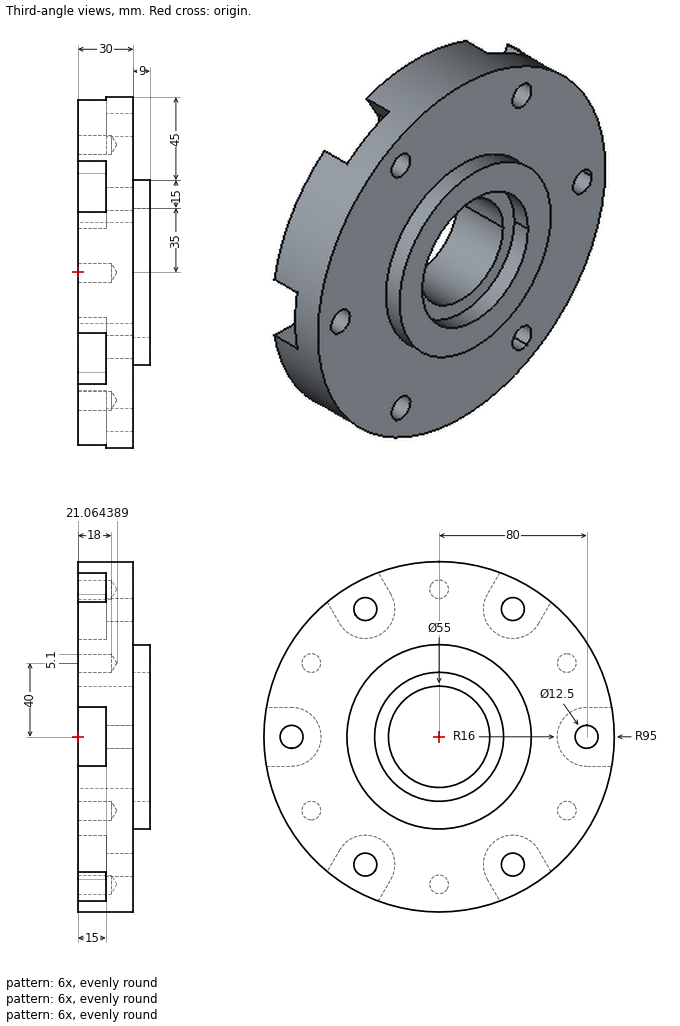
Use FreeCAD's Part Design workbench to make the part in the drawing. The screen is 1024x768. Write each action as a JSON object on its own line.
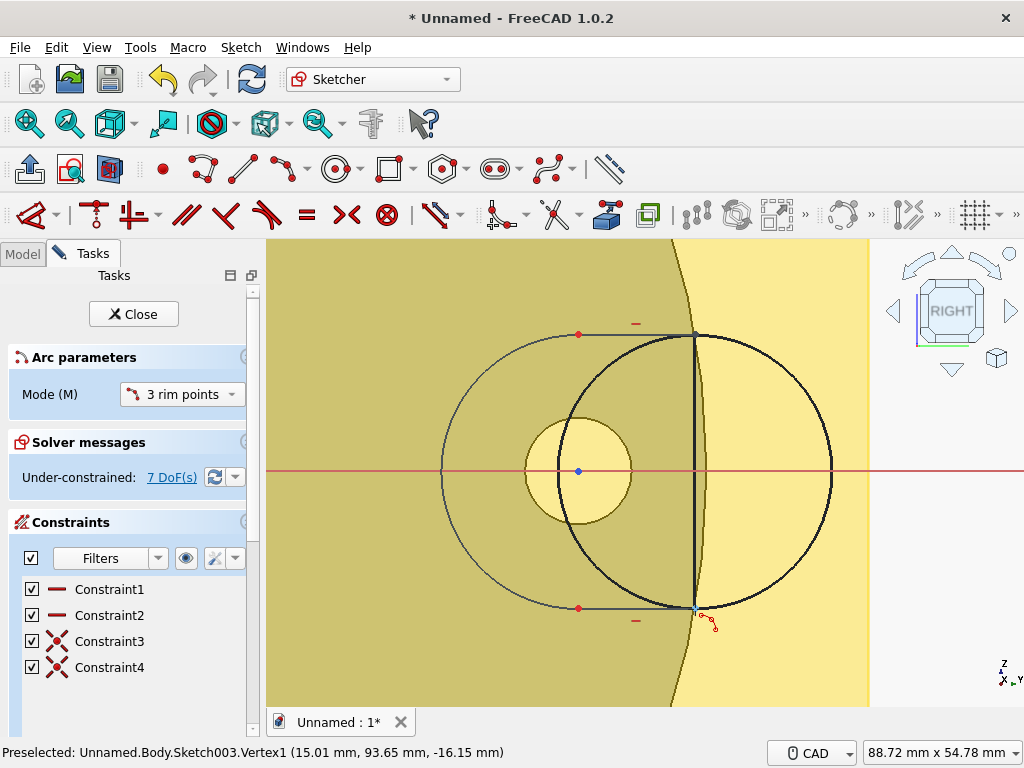
{"action": "scroll", "coordinate": [706, 498], "scroll_direction": "up", "scroll_amount": 2}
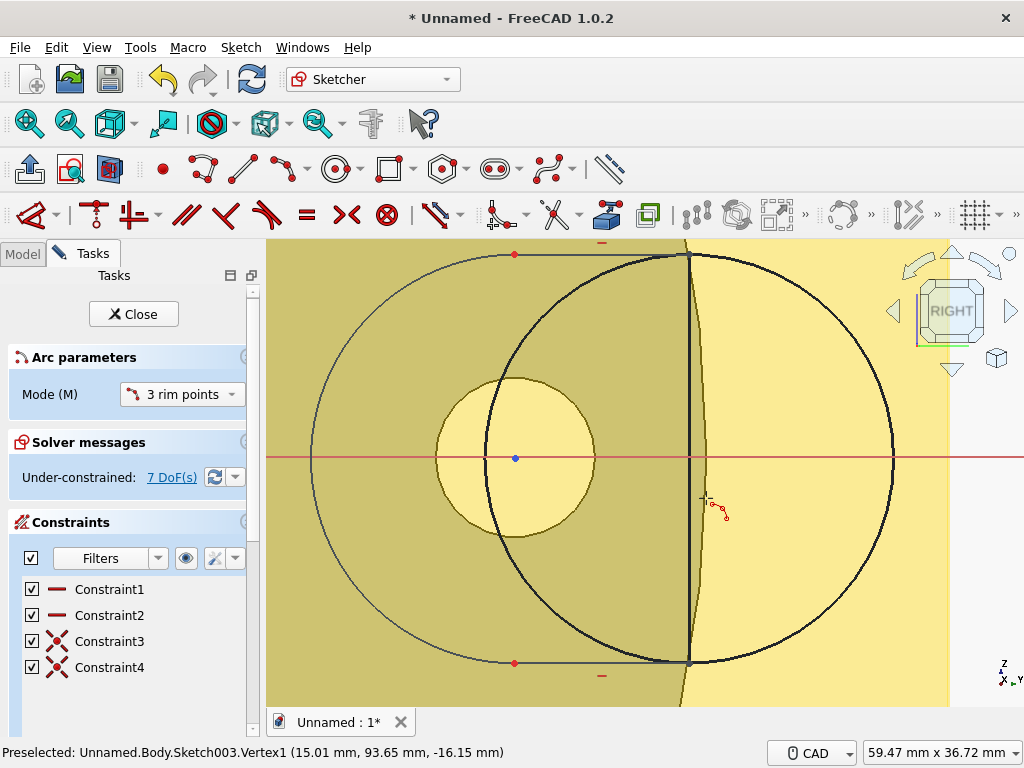
{"action": "left_click", "coordinate": [706, 498]}
{"action": "key", "text": "Escape"}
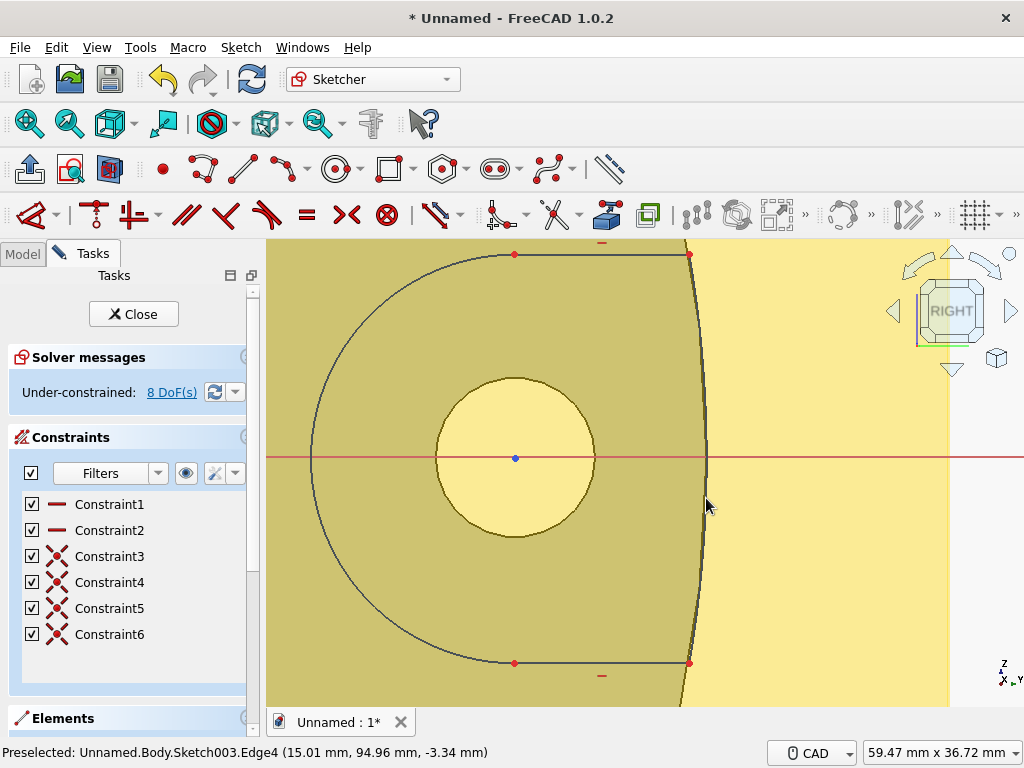
{"action": "left_click", "coordinate": [637, 663]}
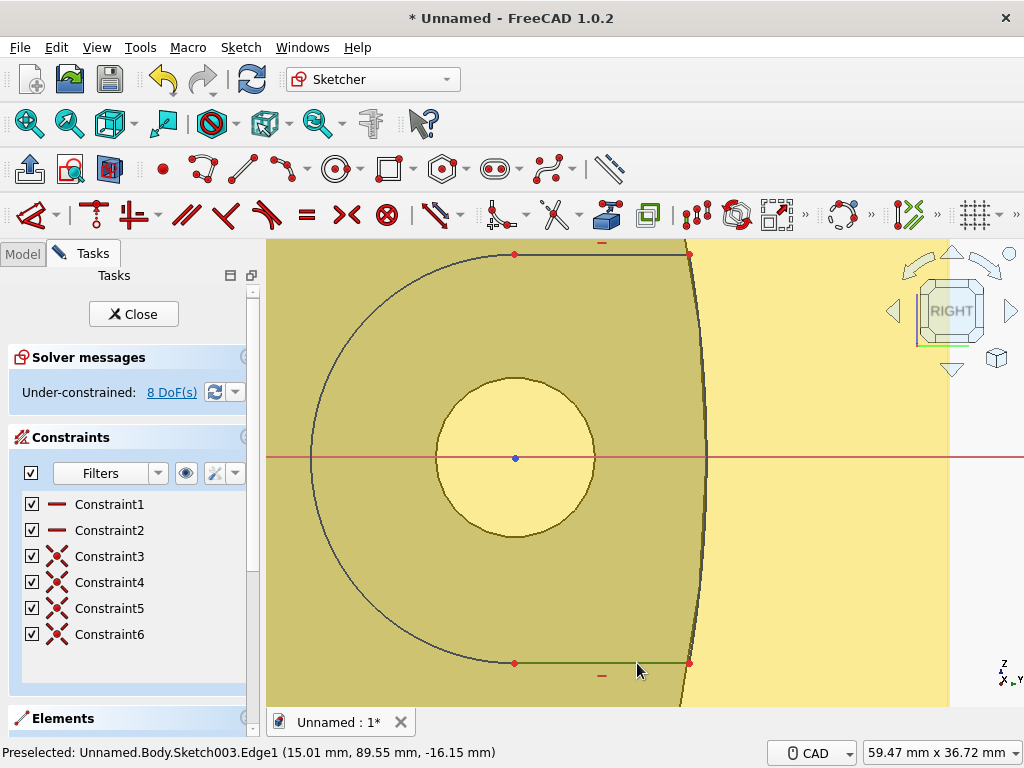
{"action": "left_click", "coordinate": [350, 339]}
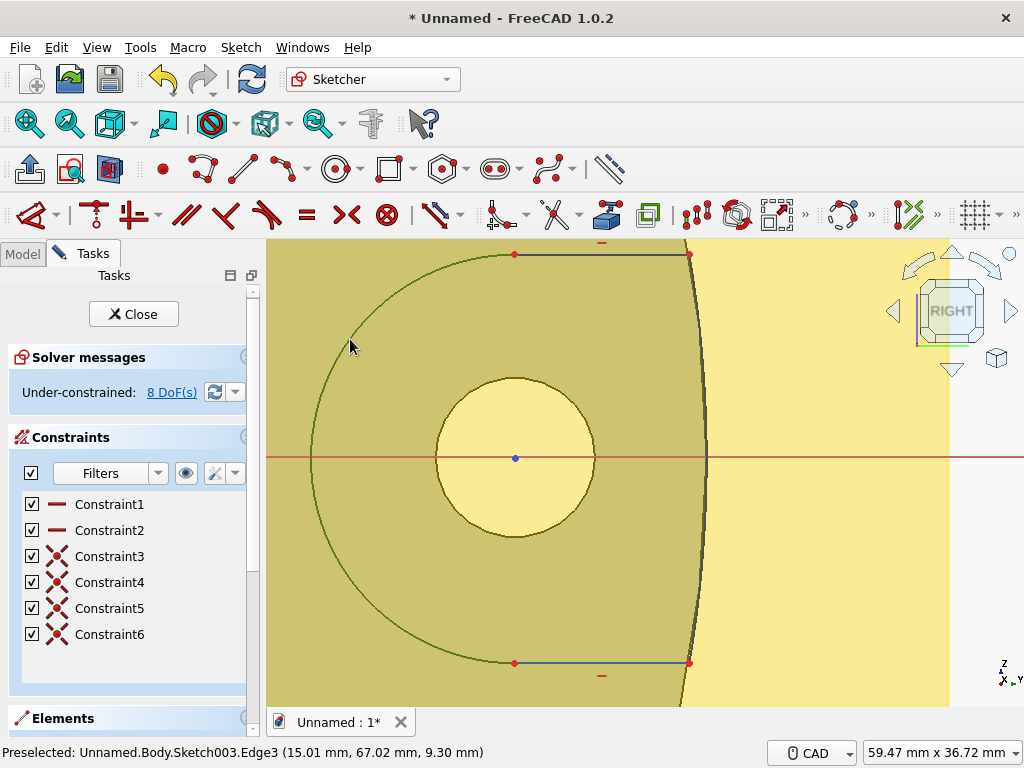
{"action": "left_click", "coordinate": [268, 216]}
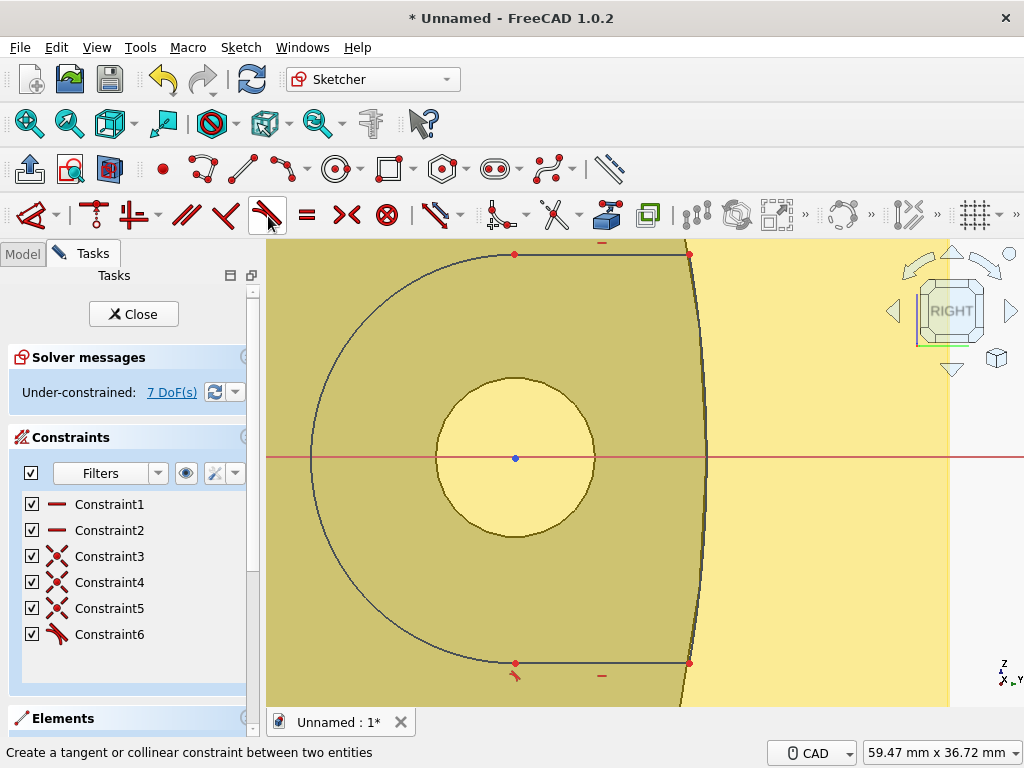
{"action": "scroll", "coordinate": [714, 505], "scroll_direction": "down", "scroll_amount": 2}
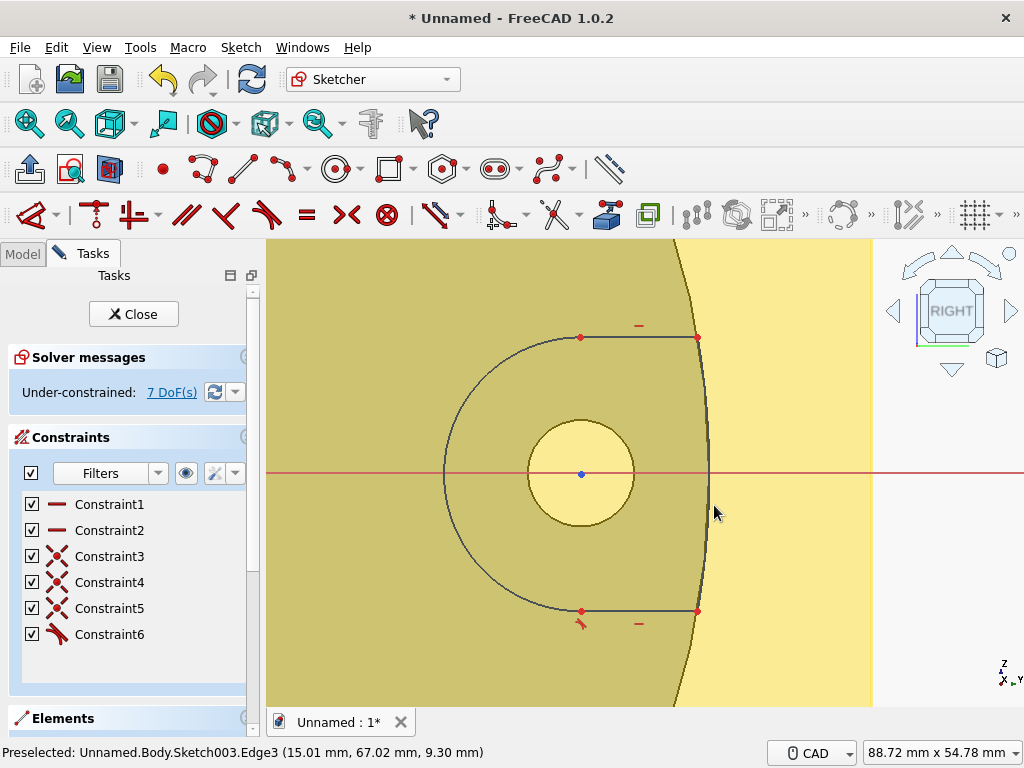
{"action": "left_click", "coordinate": [616, 337]}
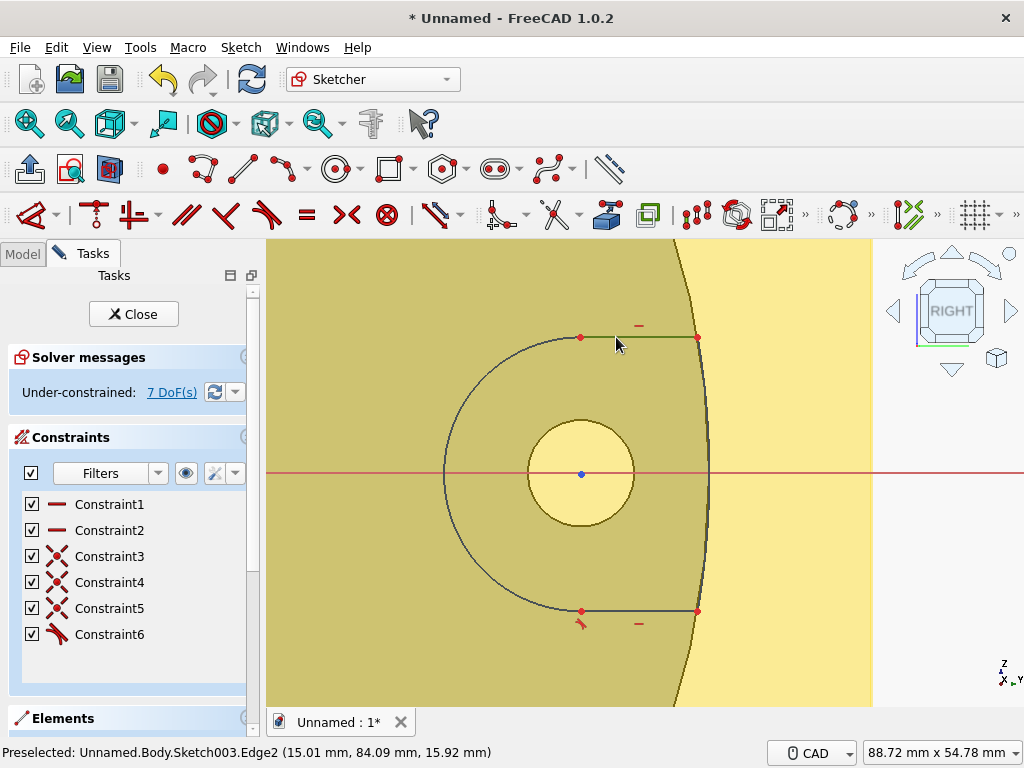
{"action": "left_click", "coordinate": [470, 394]}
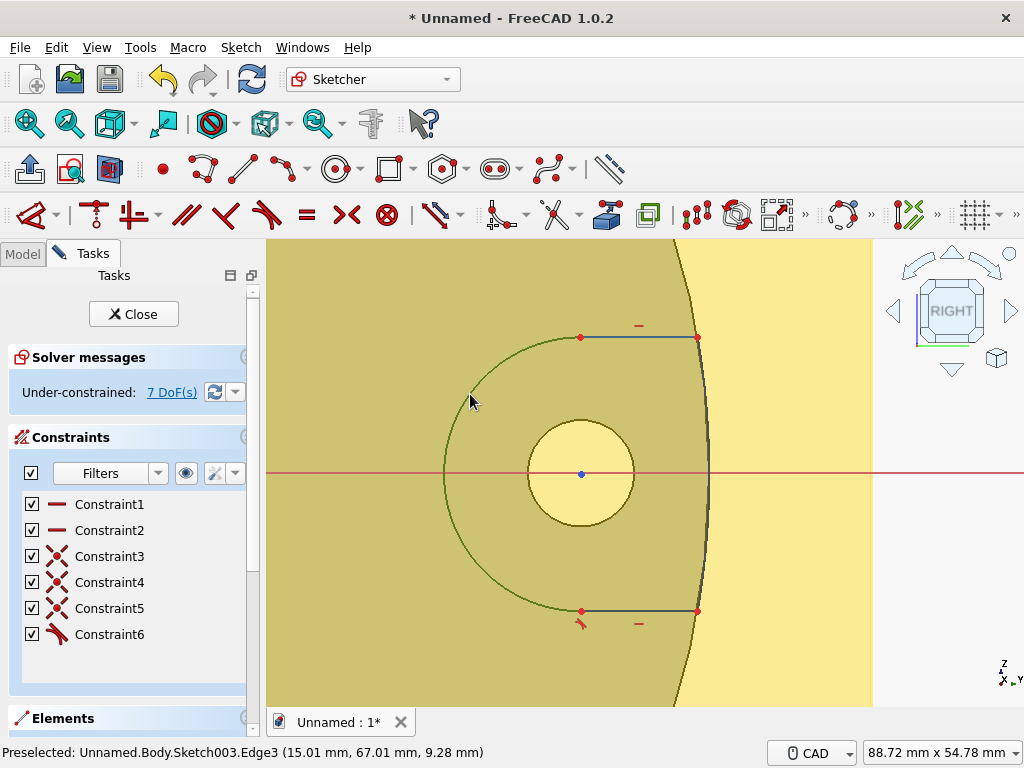
{"action": "left_click", "coordinate": [268, 216]}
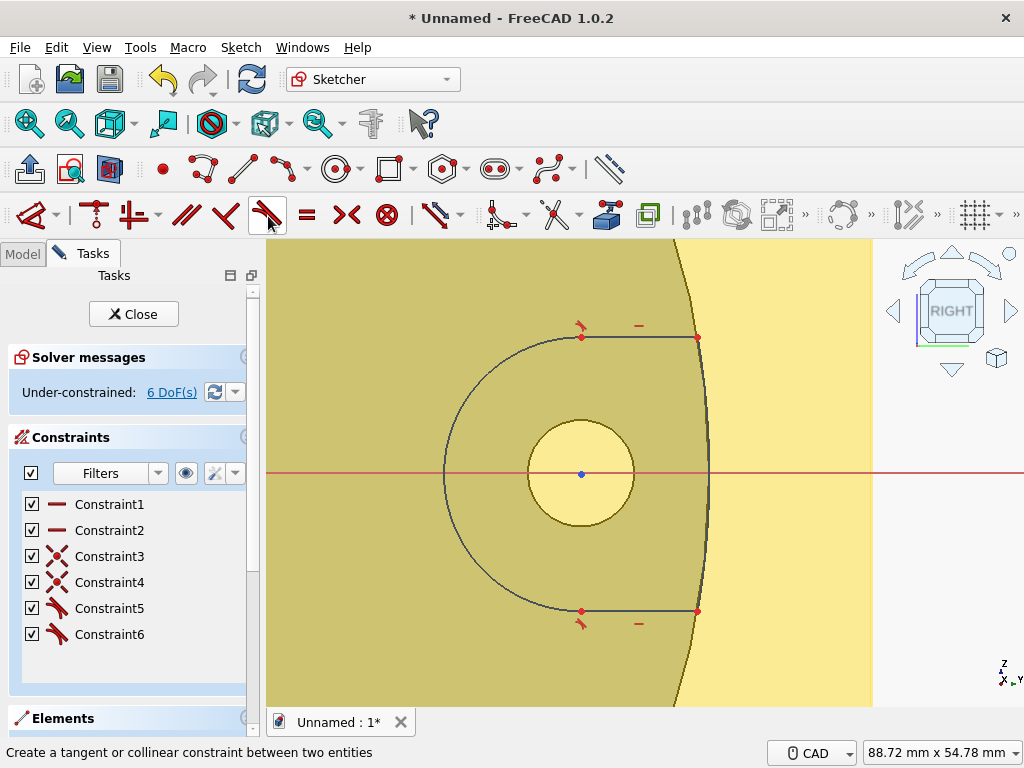
{"action": "scroll", "coordinate": [799, 473], "scroll_direction": "down", "scroll_amount": 4}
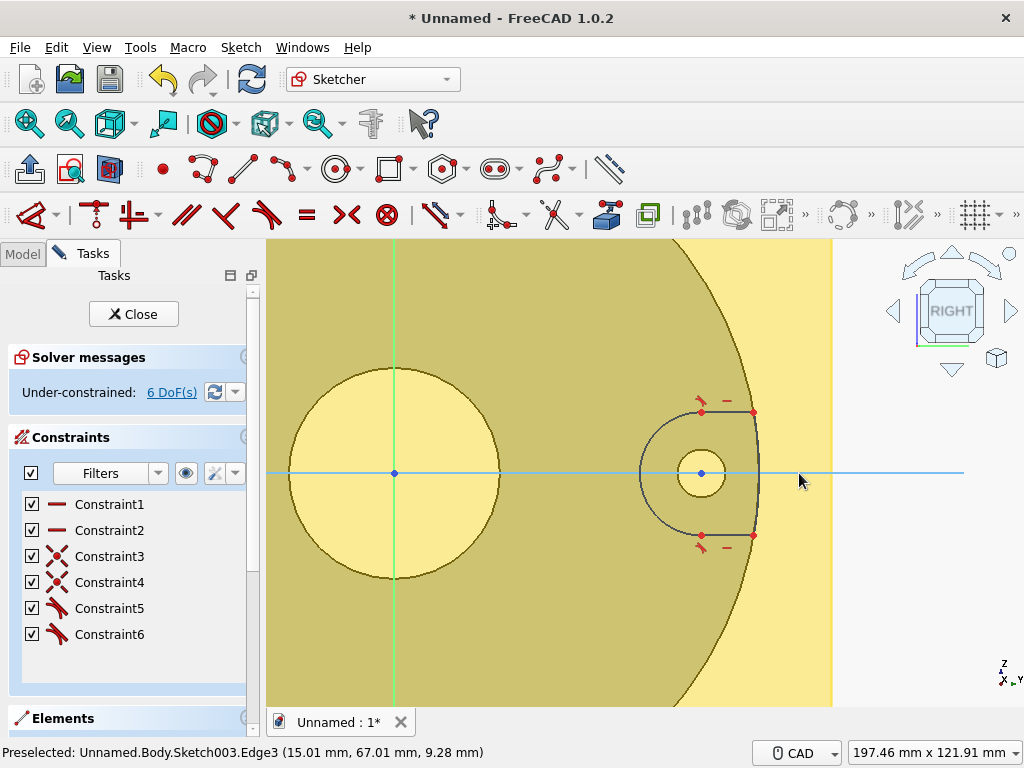
{"action": "left_click_drag", "start_coordinate": [384, 463], "coordinate": [404, 484]}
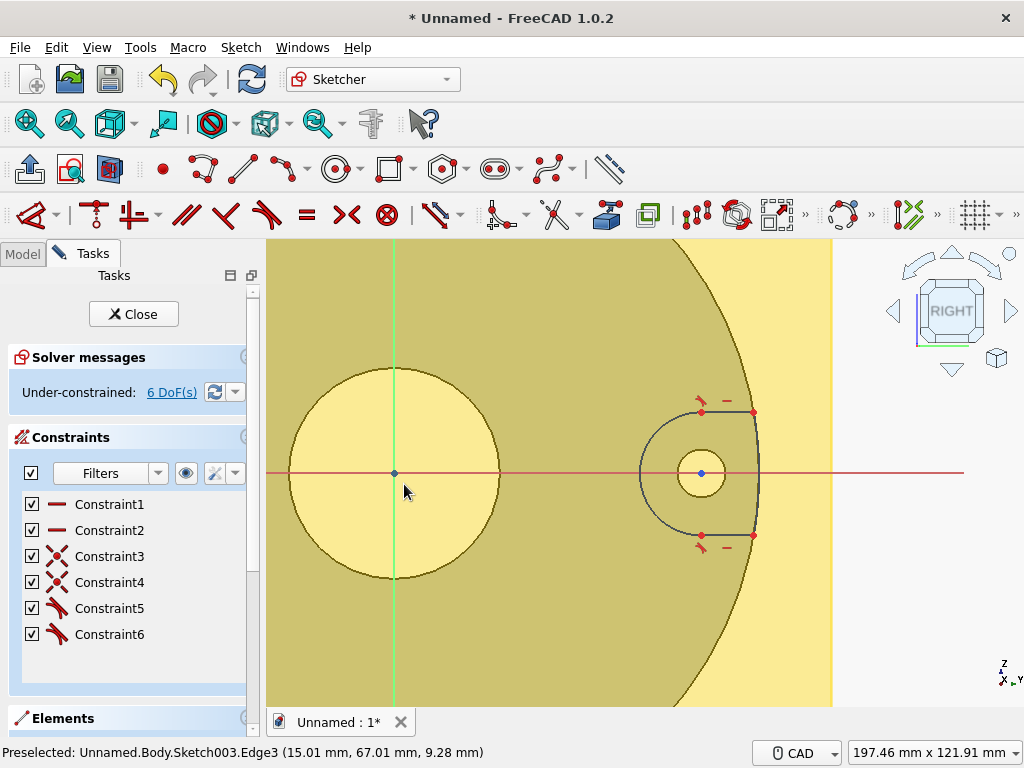
{"action": "key", "text": "c"}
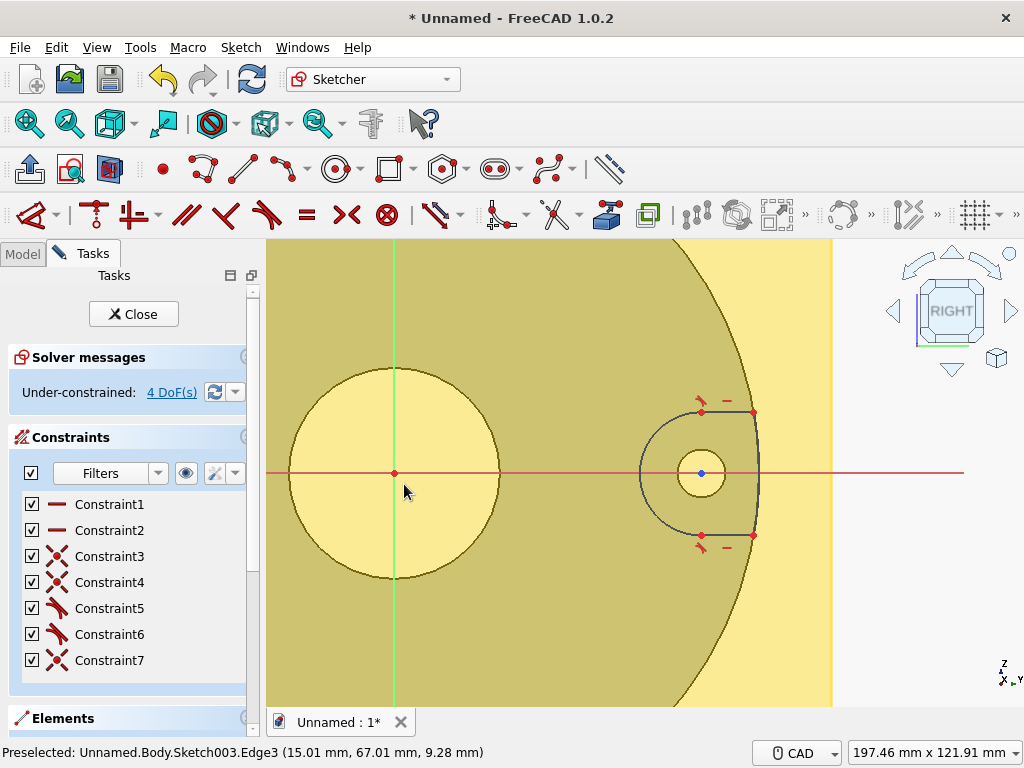
{"action": "left_click", "coordinate": [701, 474]}